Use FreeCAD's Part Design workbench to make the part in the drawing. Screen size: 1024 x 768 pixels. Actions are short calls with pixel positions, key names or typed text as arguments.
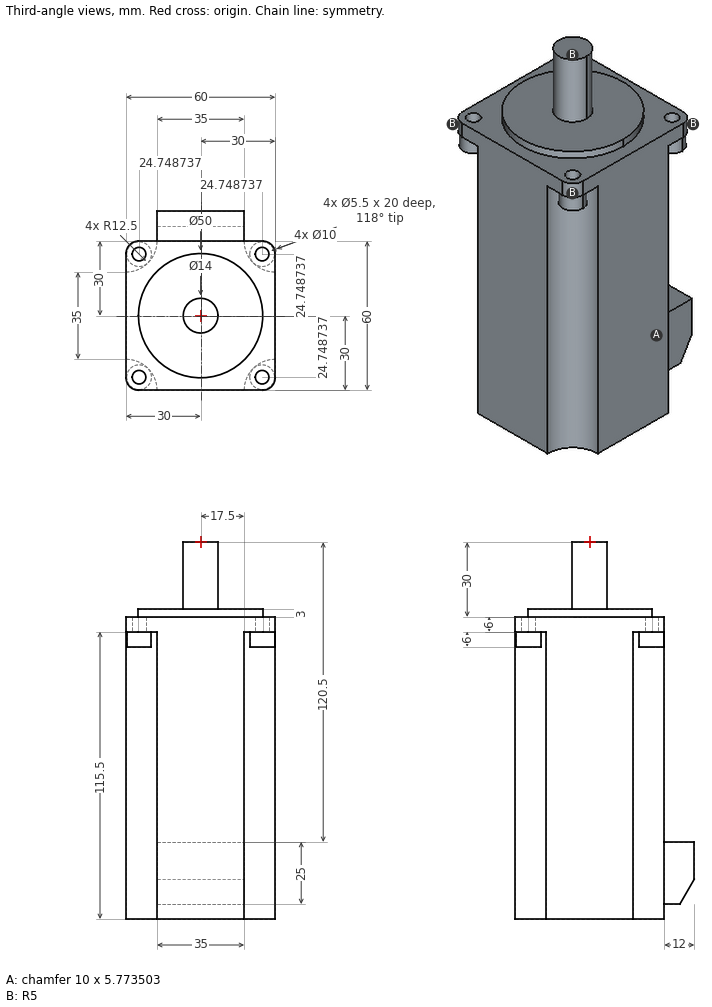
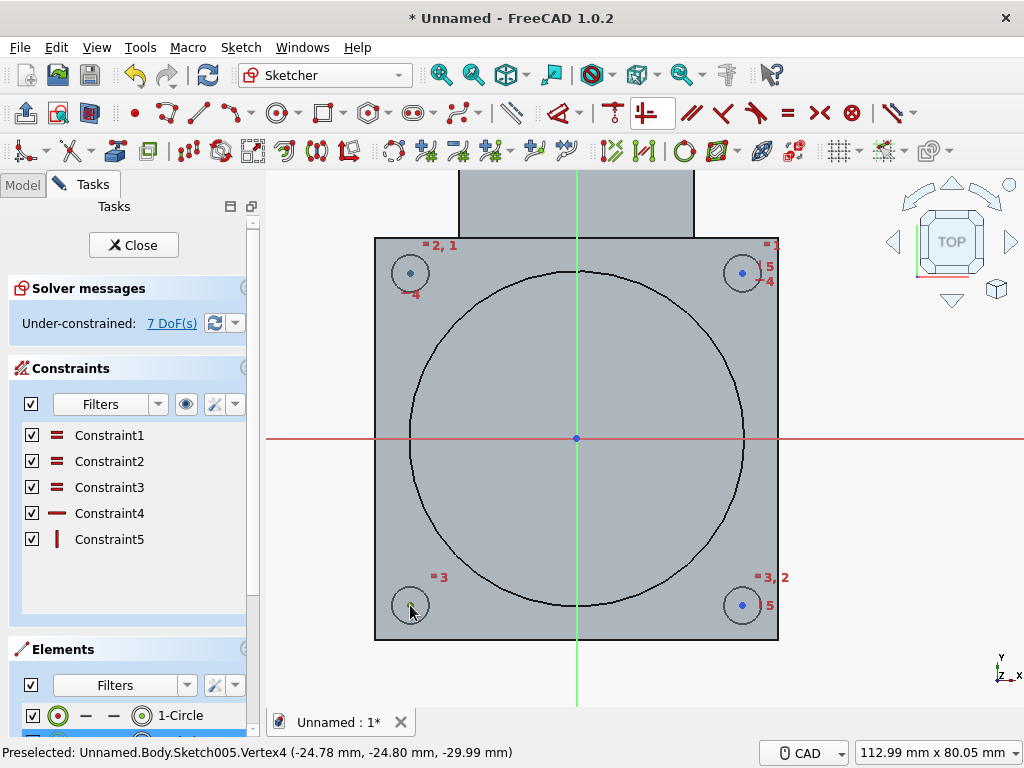
click(670, 114)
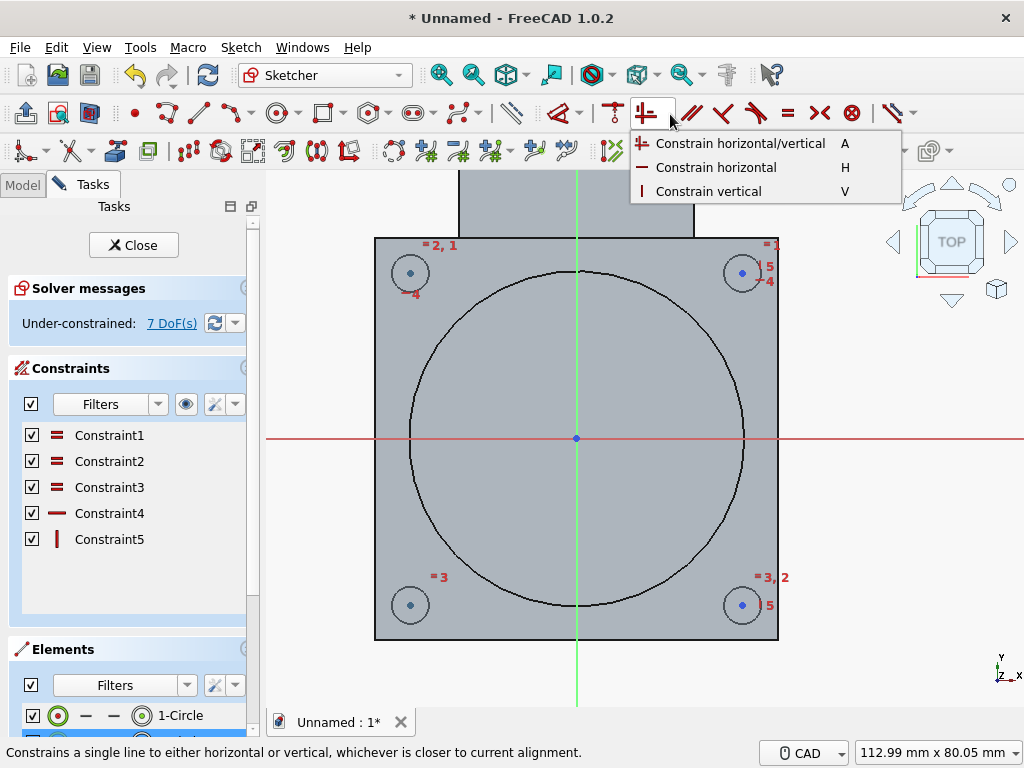
click(766, 191)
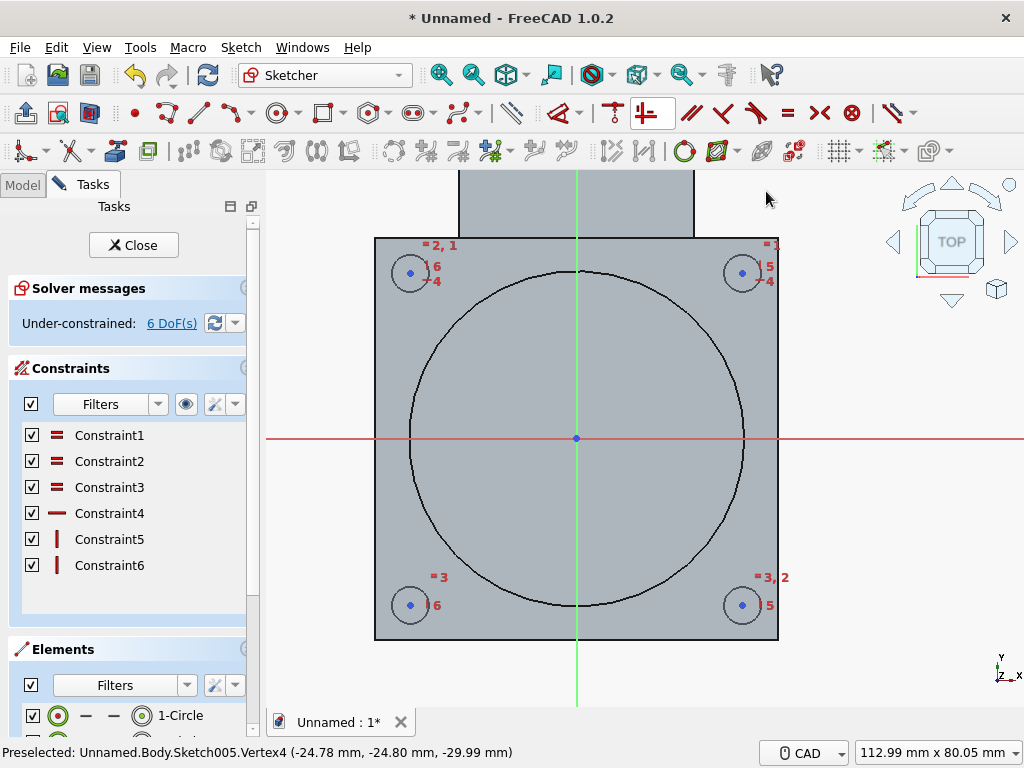
click(743, 606)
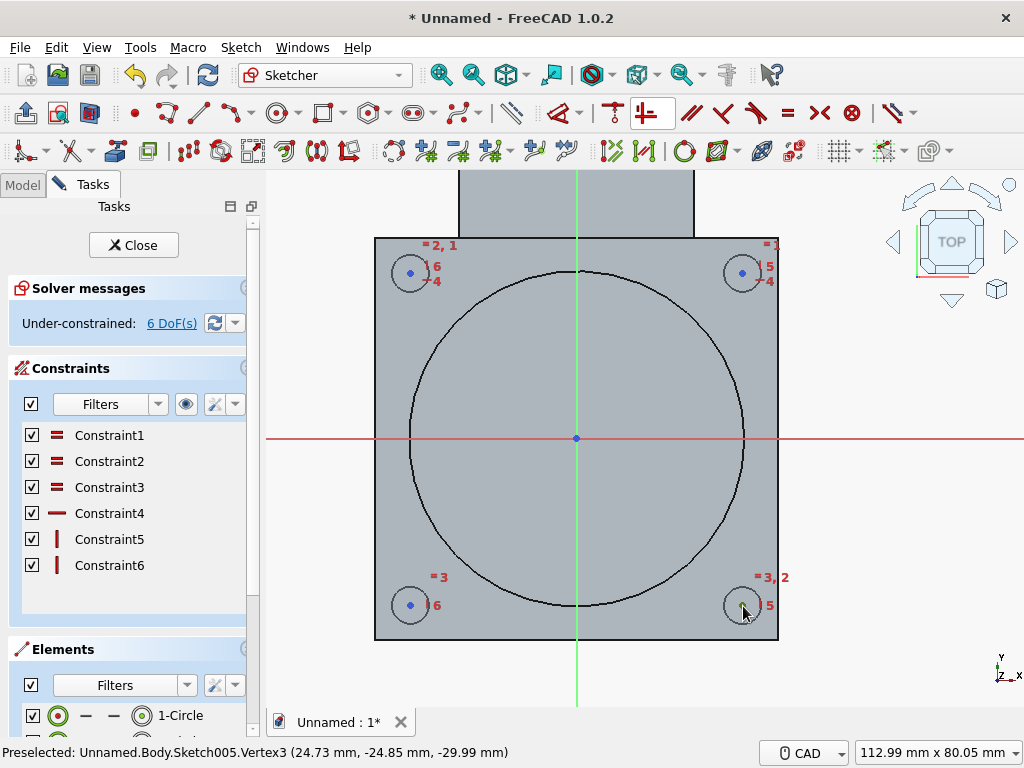
click(410, 605)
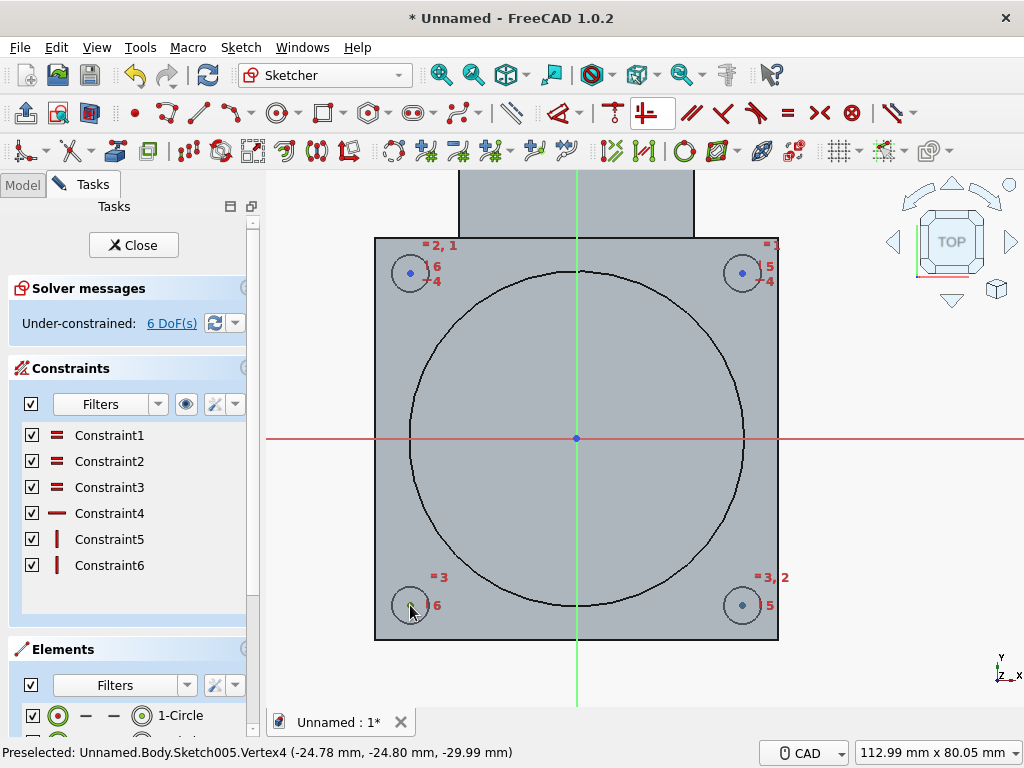
click(670, 114)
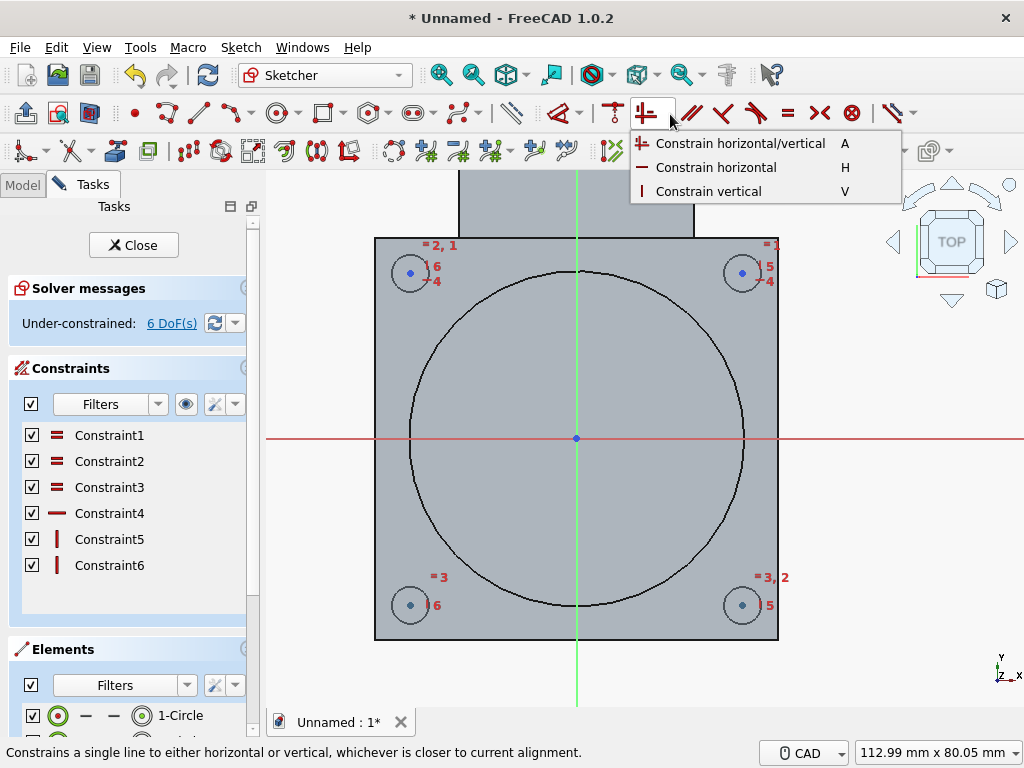
click(766, 167)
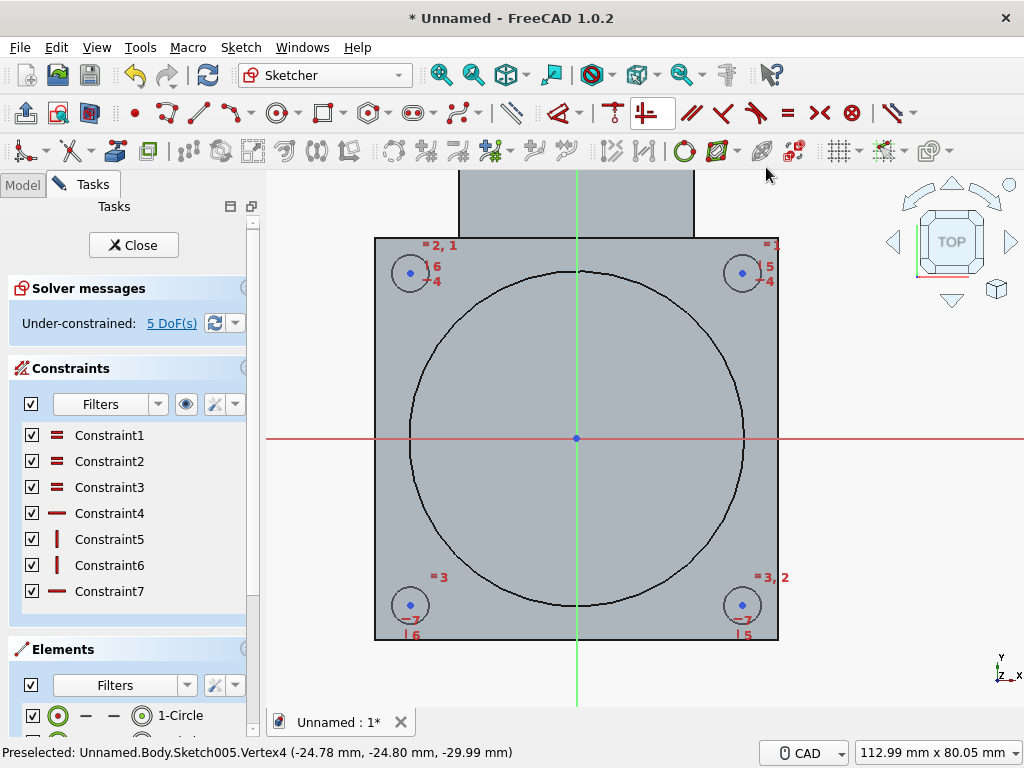
click(558, 114)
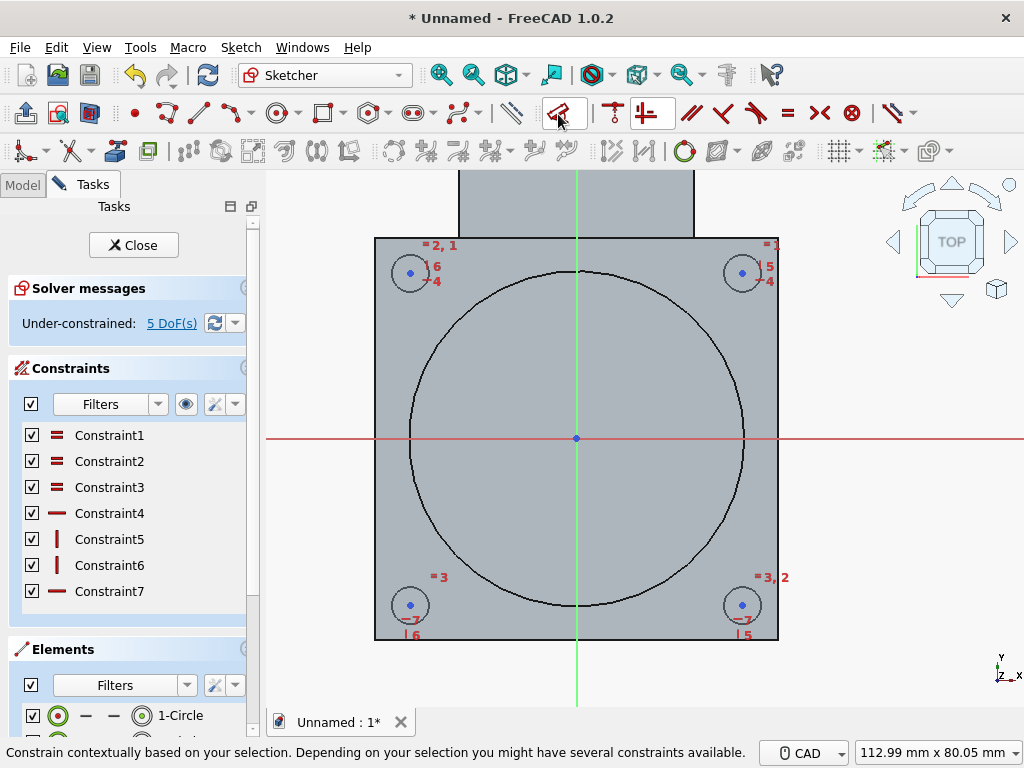
click(756, 260)
click(779, 237)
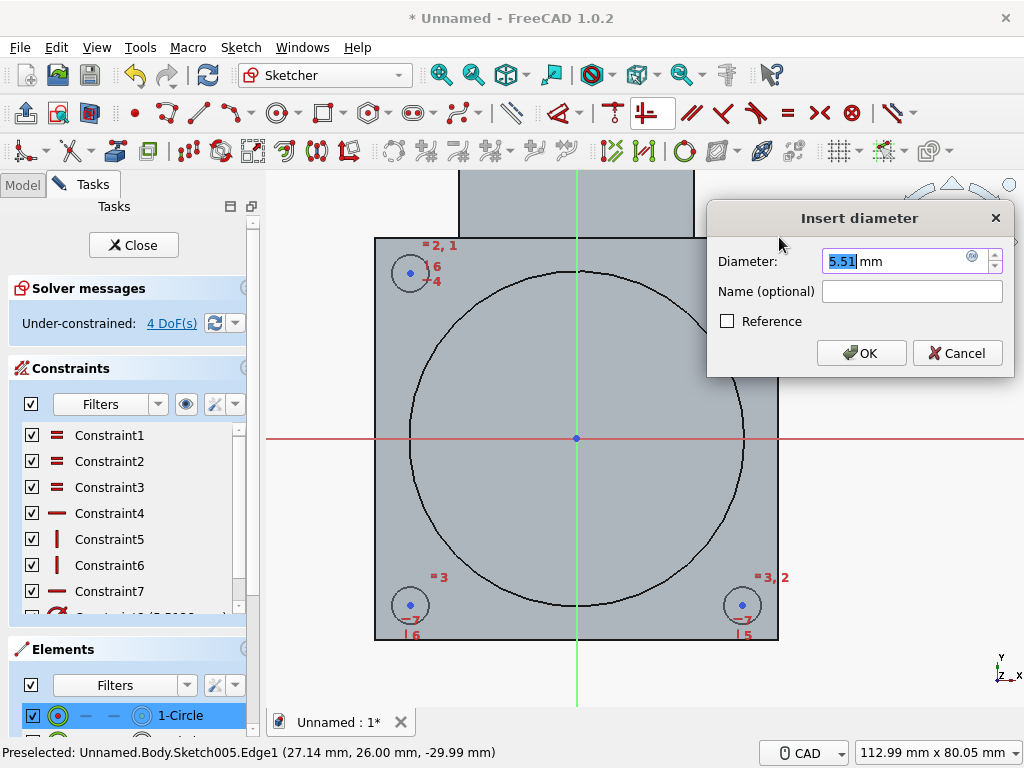
text(5.5)
key(Return)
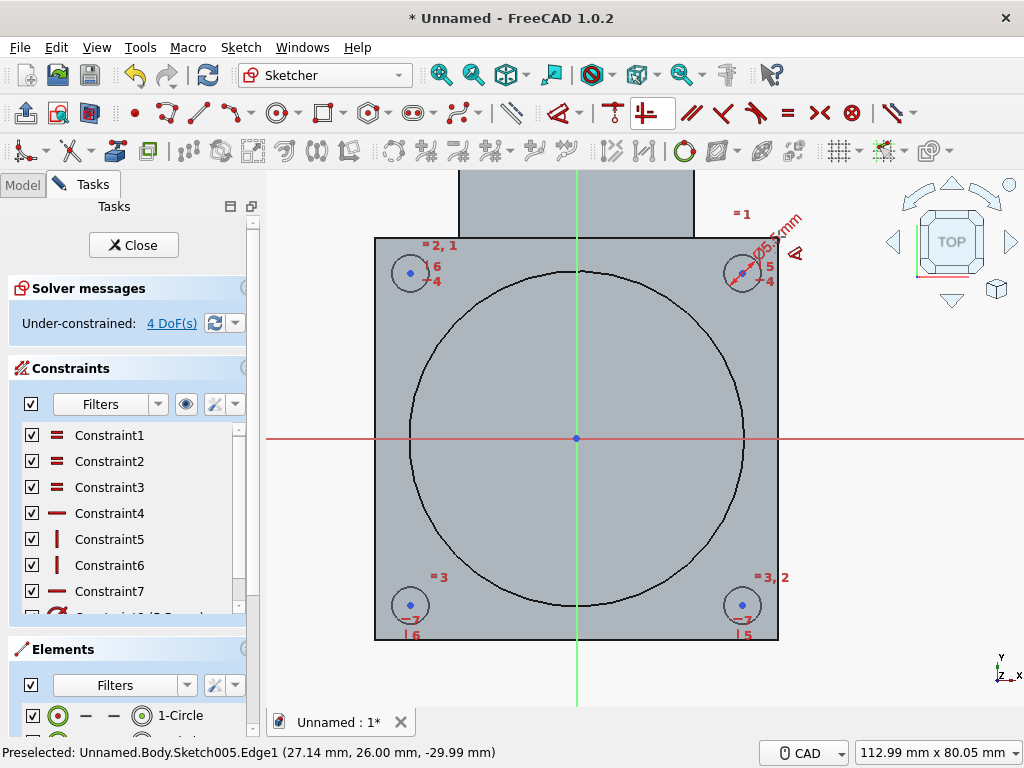
click(743, 273)
click(660, 239)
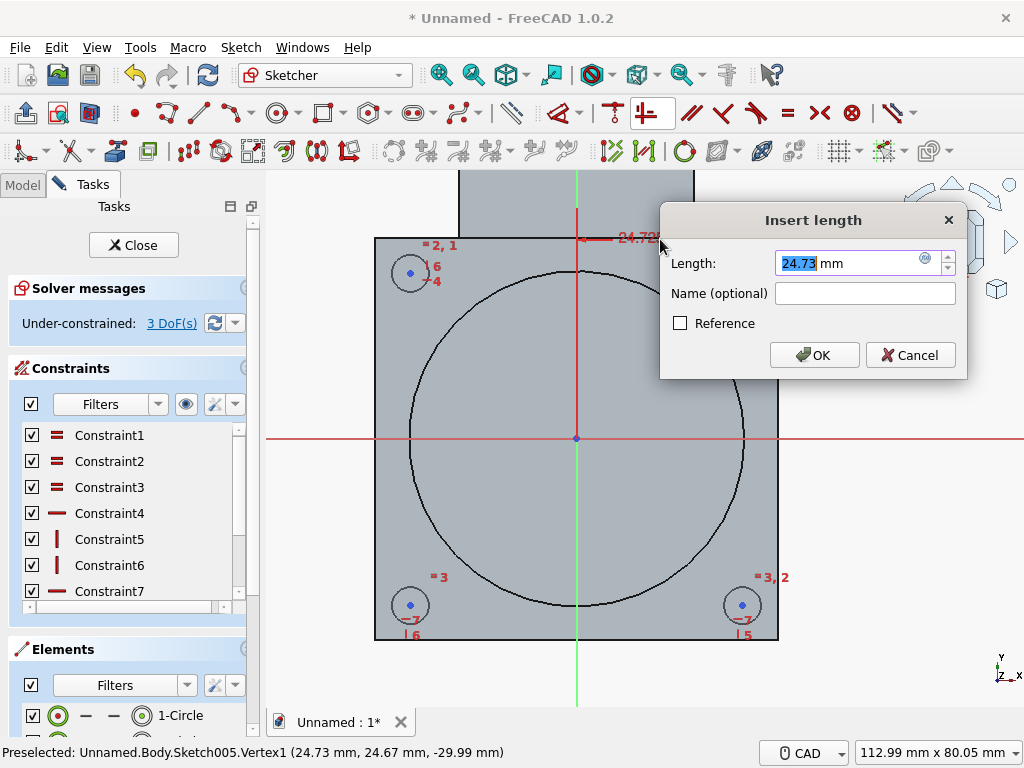
text(24.748737)
key(Return)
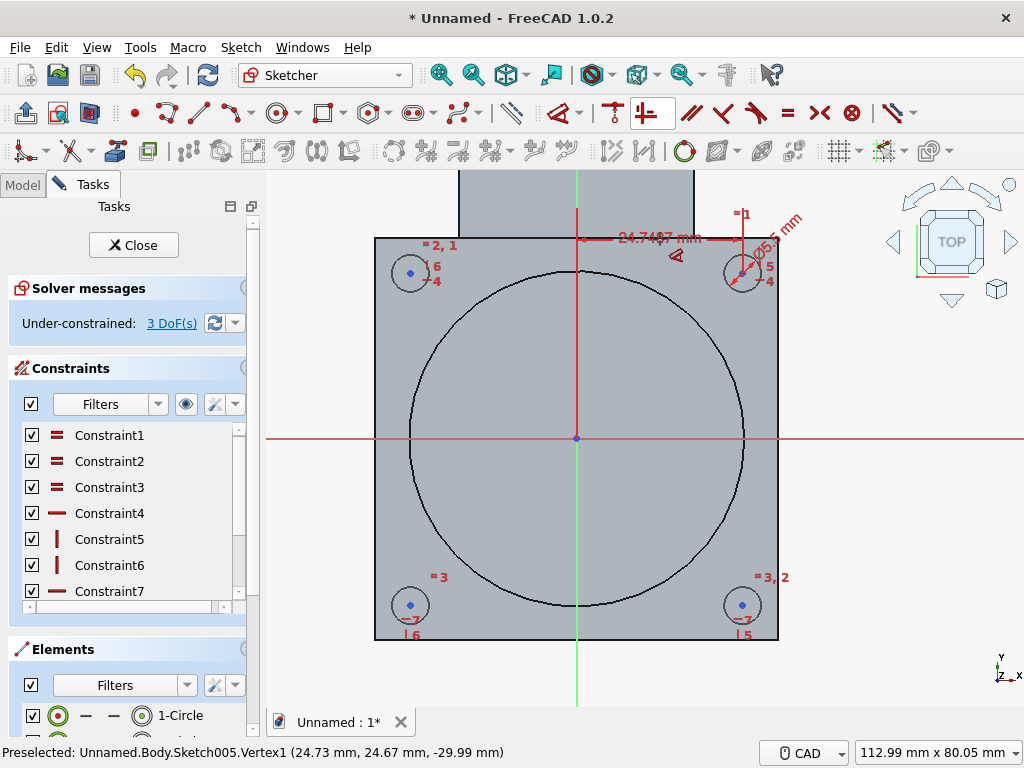
click(743, 273)
click(777, 356)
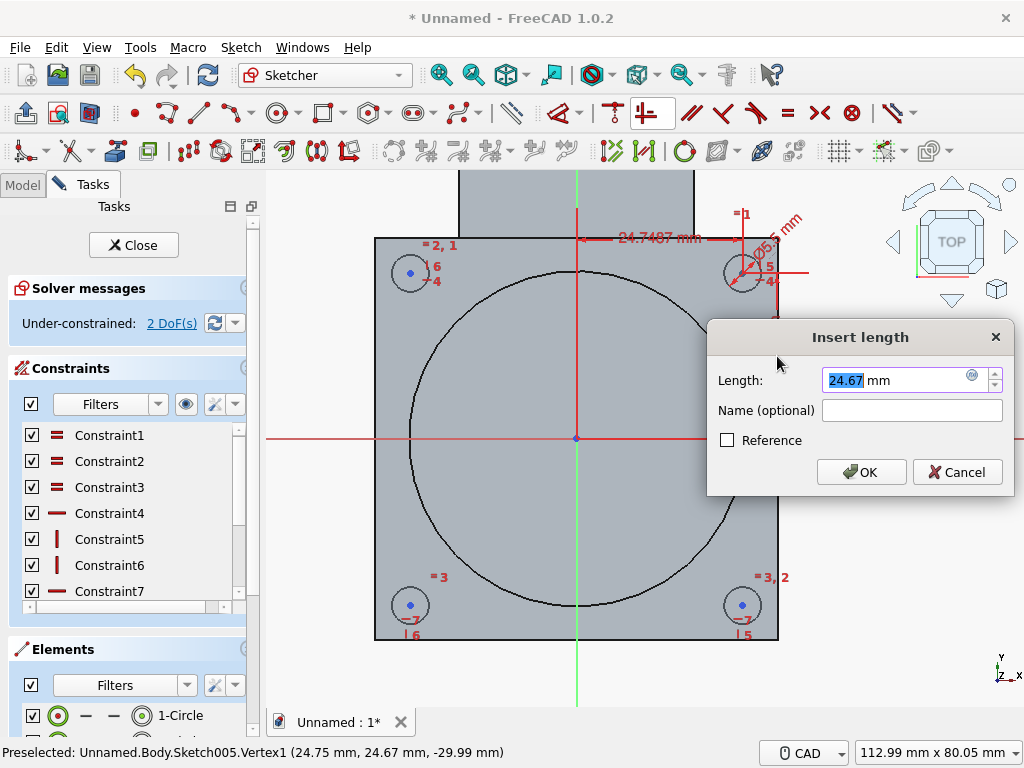
text(24.748737)
key(Return)